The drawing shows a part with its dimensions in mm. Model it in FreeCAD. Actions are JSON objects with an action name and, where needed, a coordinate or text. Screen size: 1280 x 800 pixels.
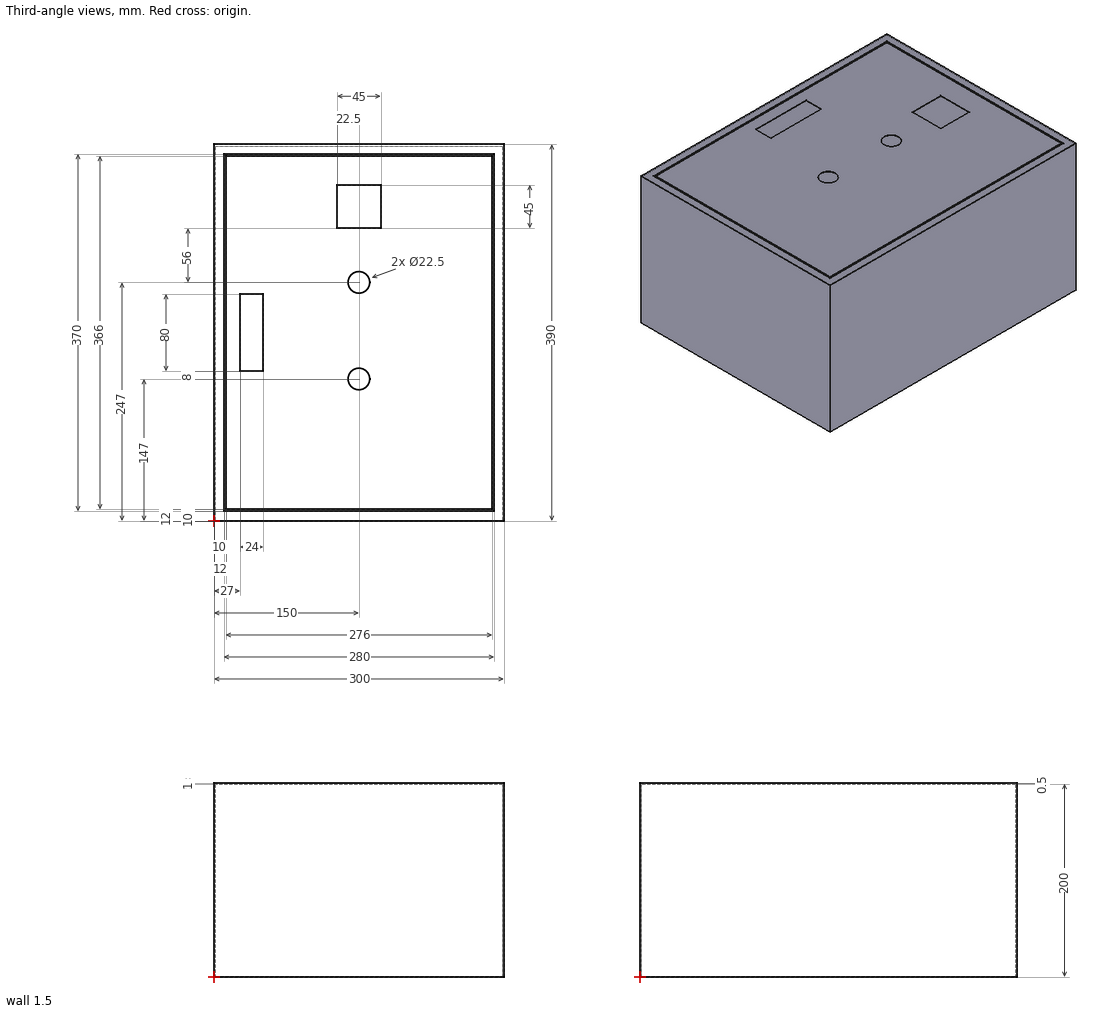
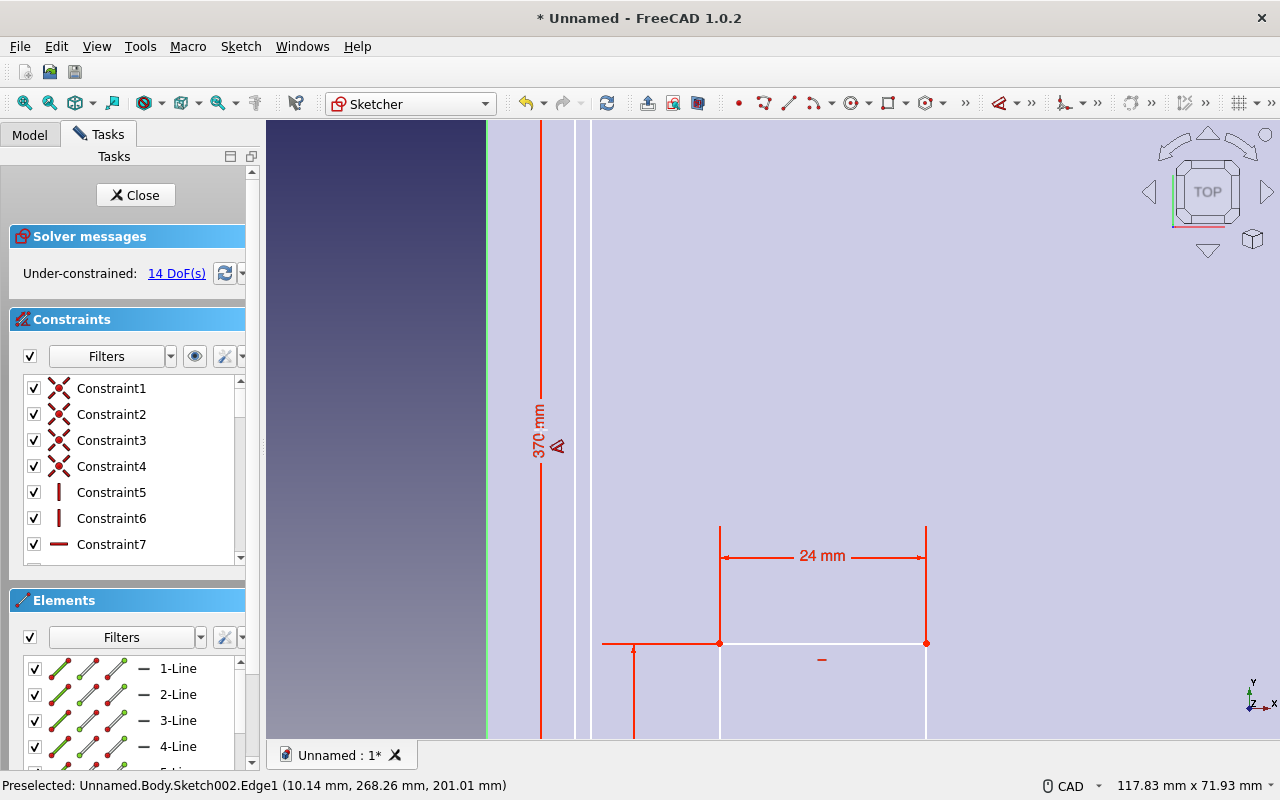
{"action": "scroll", "coordinate": [576, 355], "scroll_direction": "down", "scroll_amount": 11}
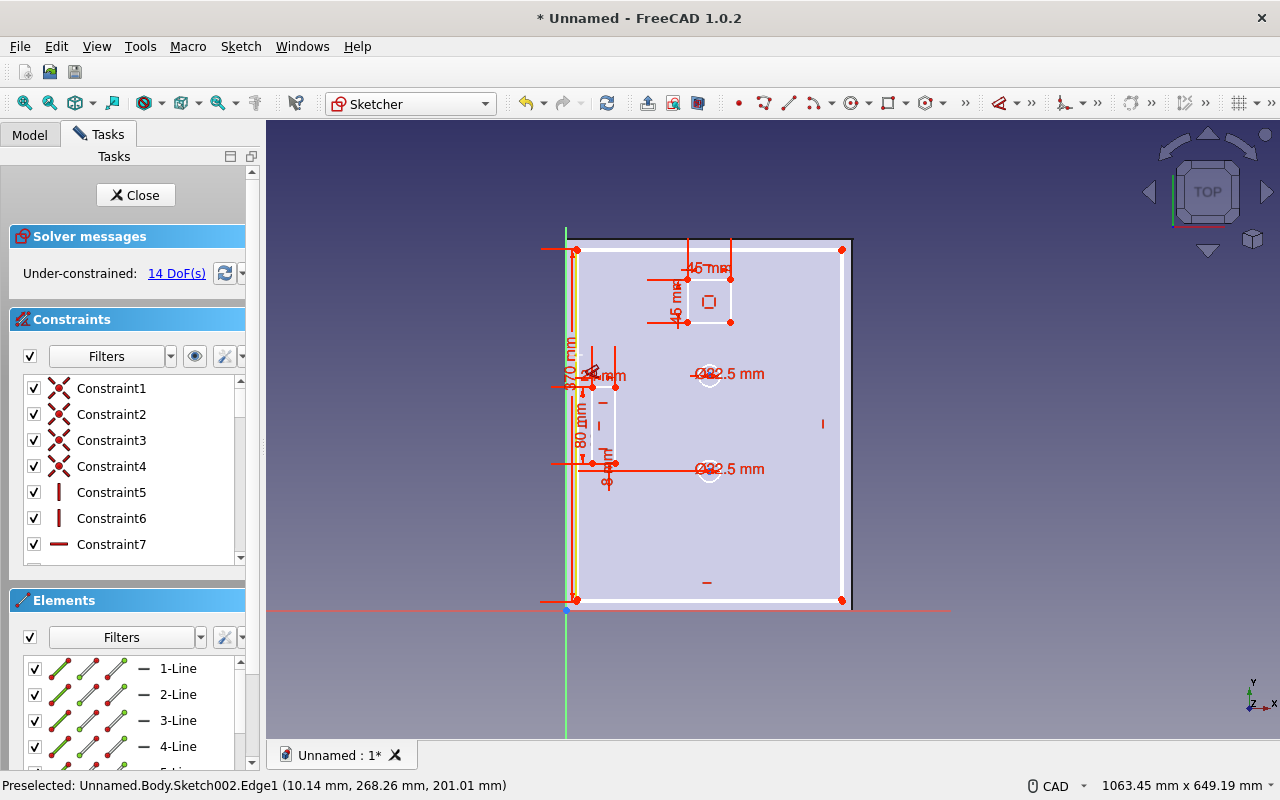
{"action": "scroll", "coordinate": [656, 602], "scroll_direction": "up", "scroll_amount": 9}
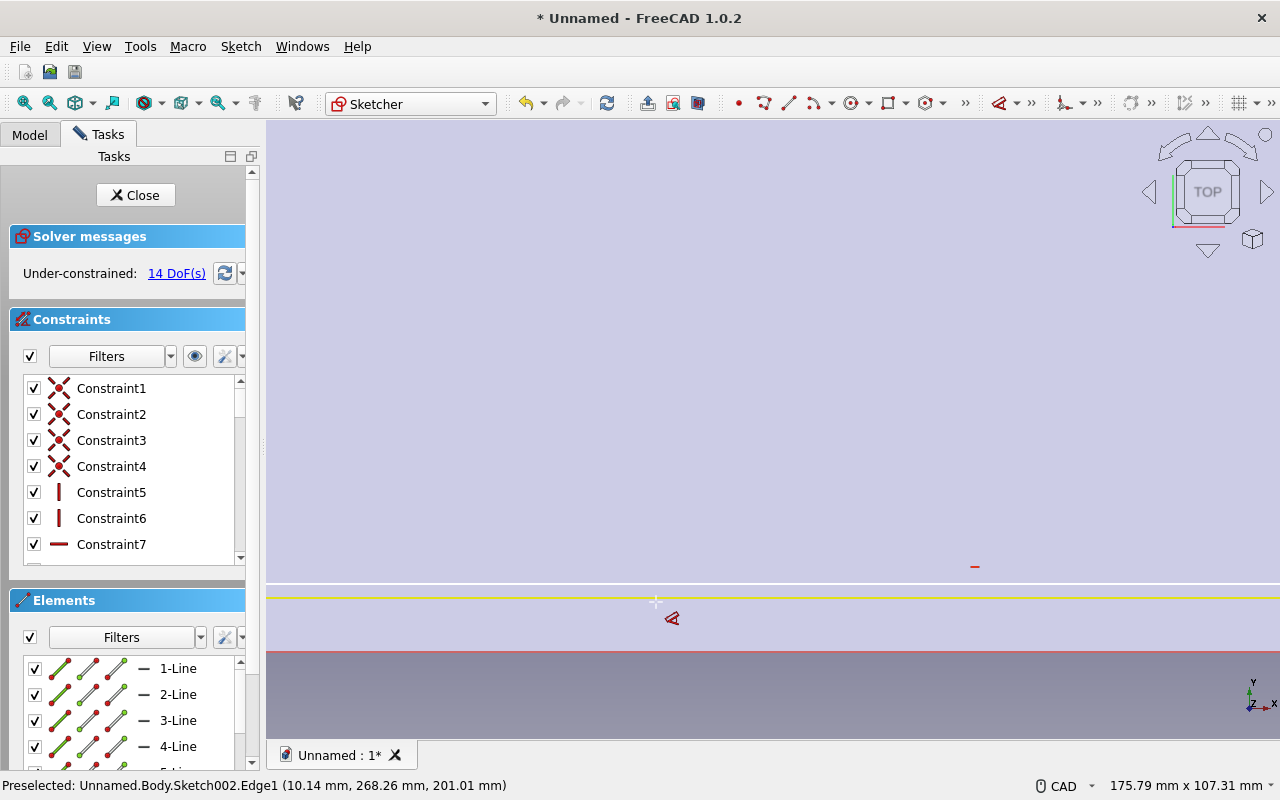
{"action": "left_click", "coordinate": [655, 598]}
{"action": "left_click", "coordinate": [704, 632]}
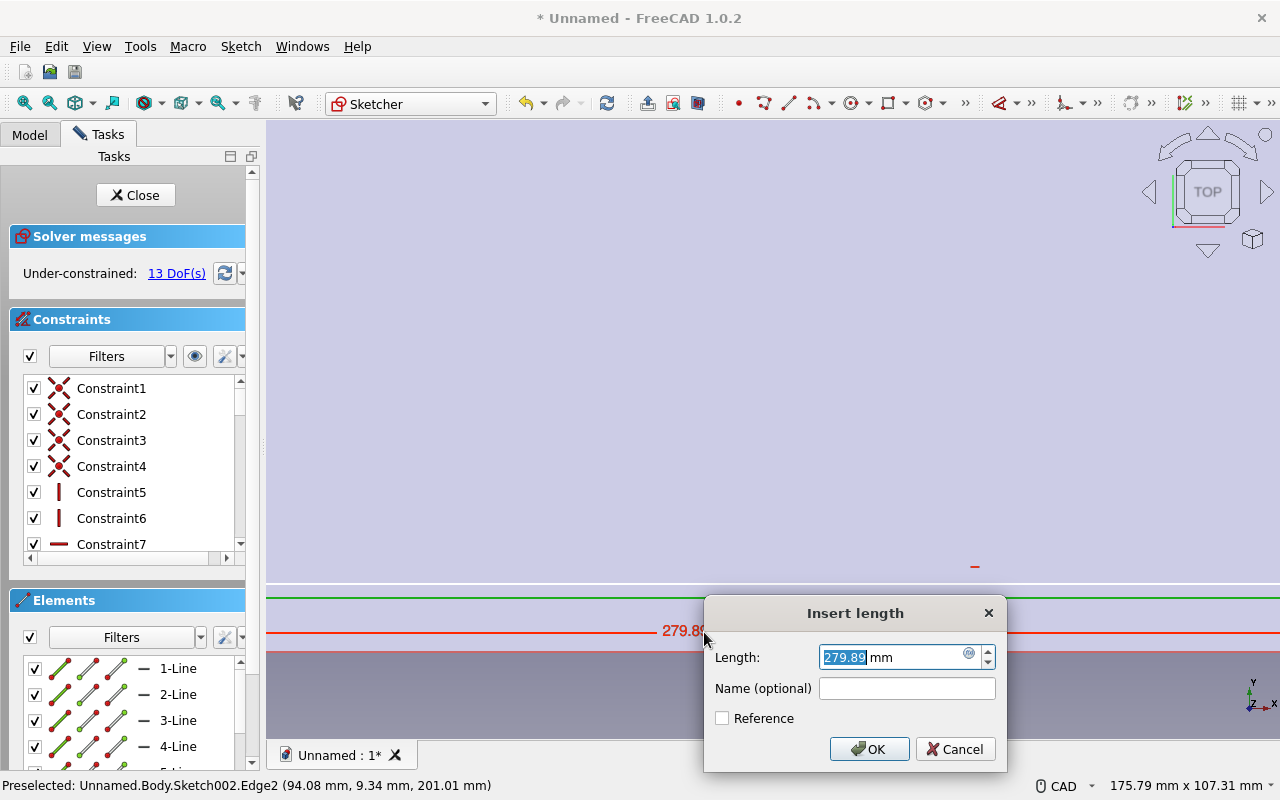
{"action": "type", "text": "280"}
{"action": "key", "text": "Return"}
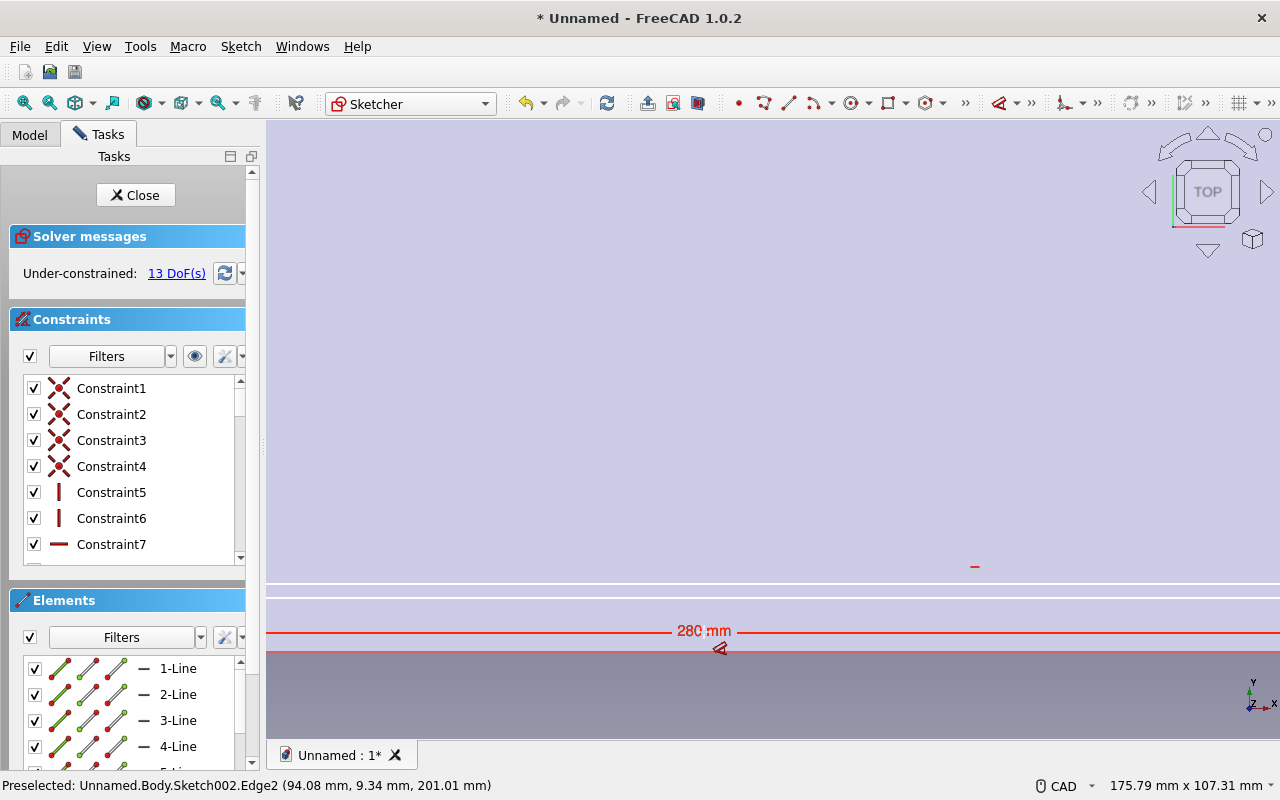
{"action": "scroll", "coordinate": [656, 603], "scroll_direction": "down", "scroll_amount": 9}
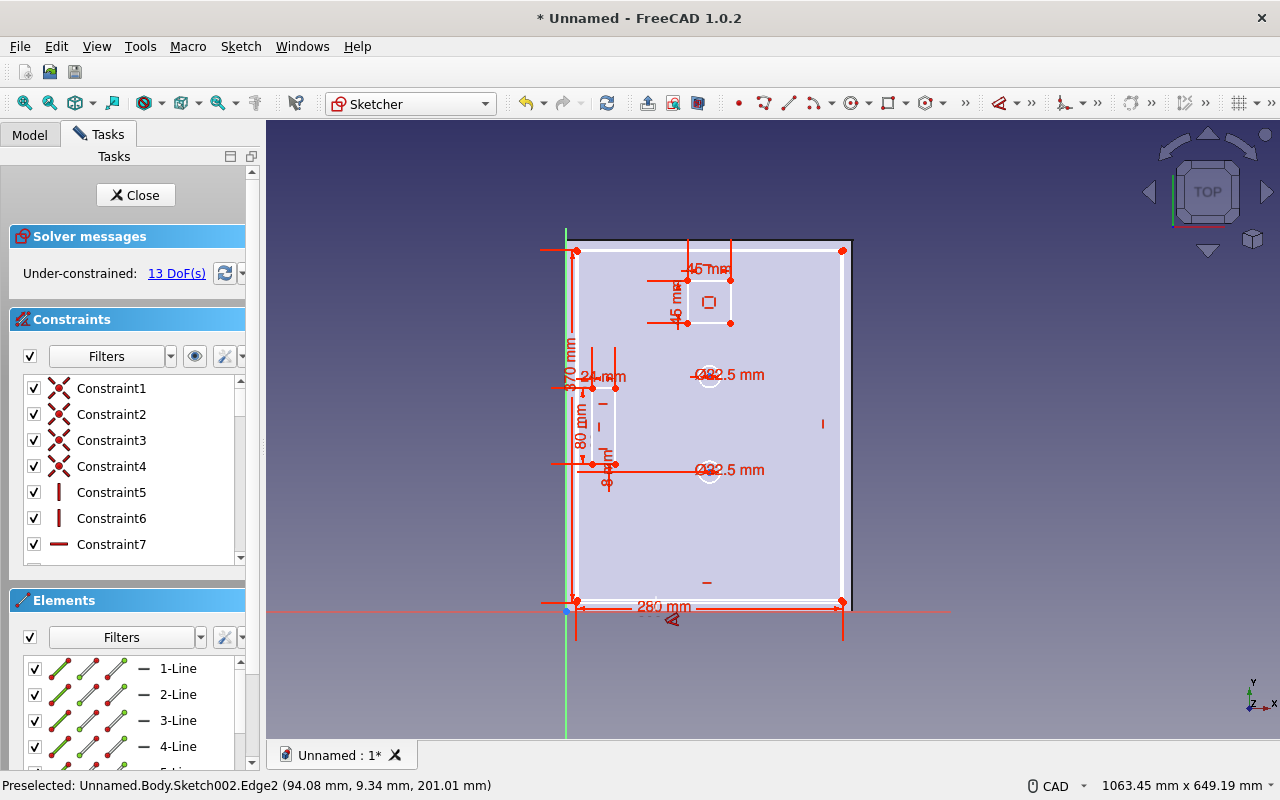
{"action": "scroll", "coordinate": [578, 356], "scroll_direction": "up", "scroll_amount": 11}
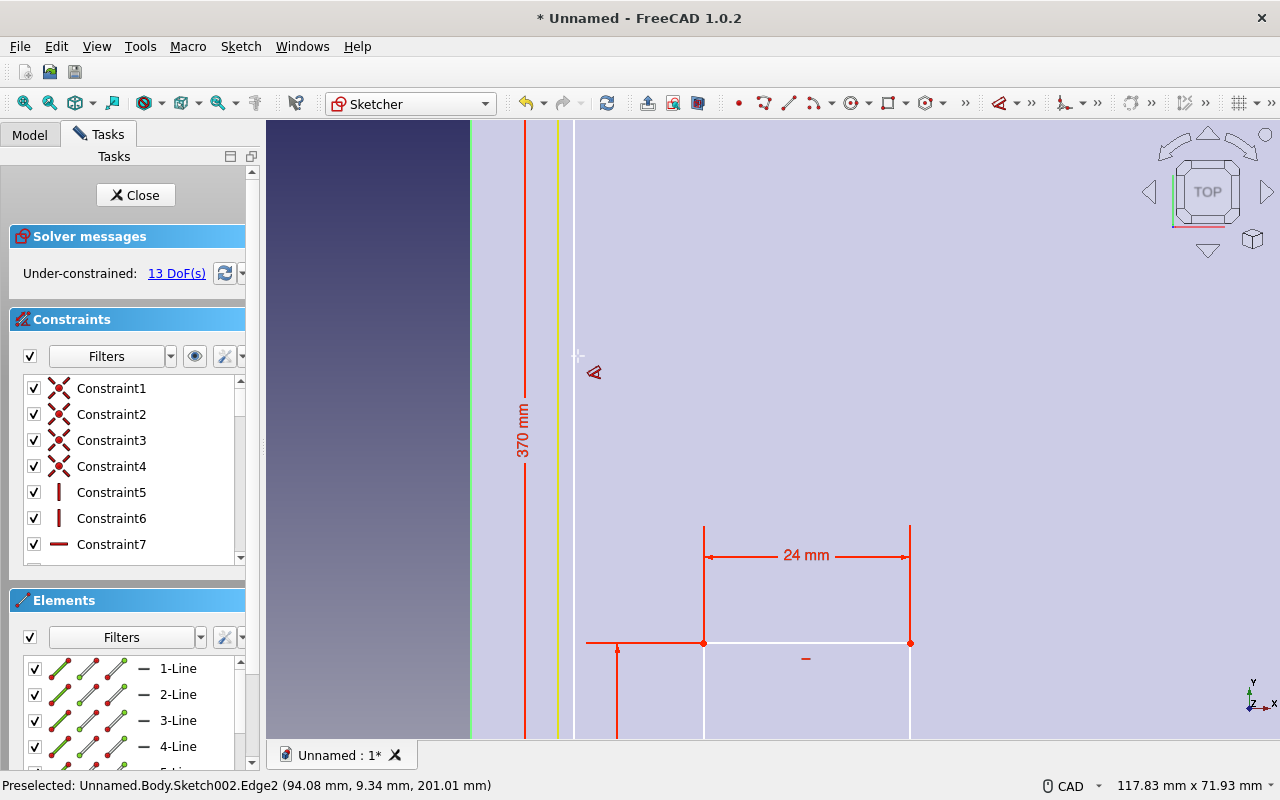
{"action": "left_click", "coordinate": [574, 354]}
{"action": "left_click", "coordinate": [540, 300]}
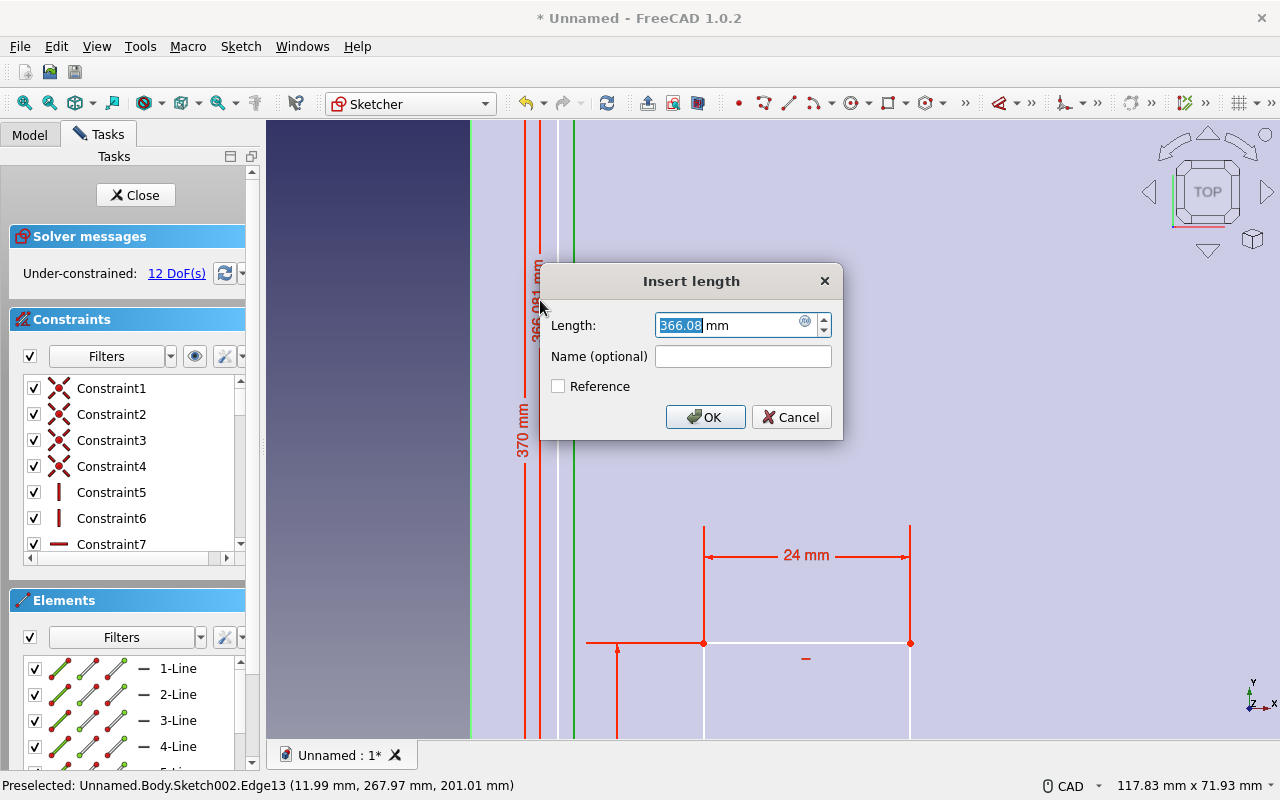
{"action": "type", "text": "366"}
{"action": "key", "text": "Return"}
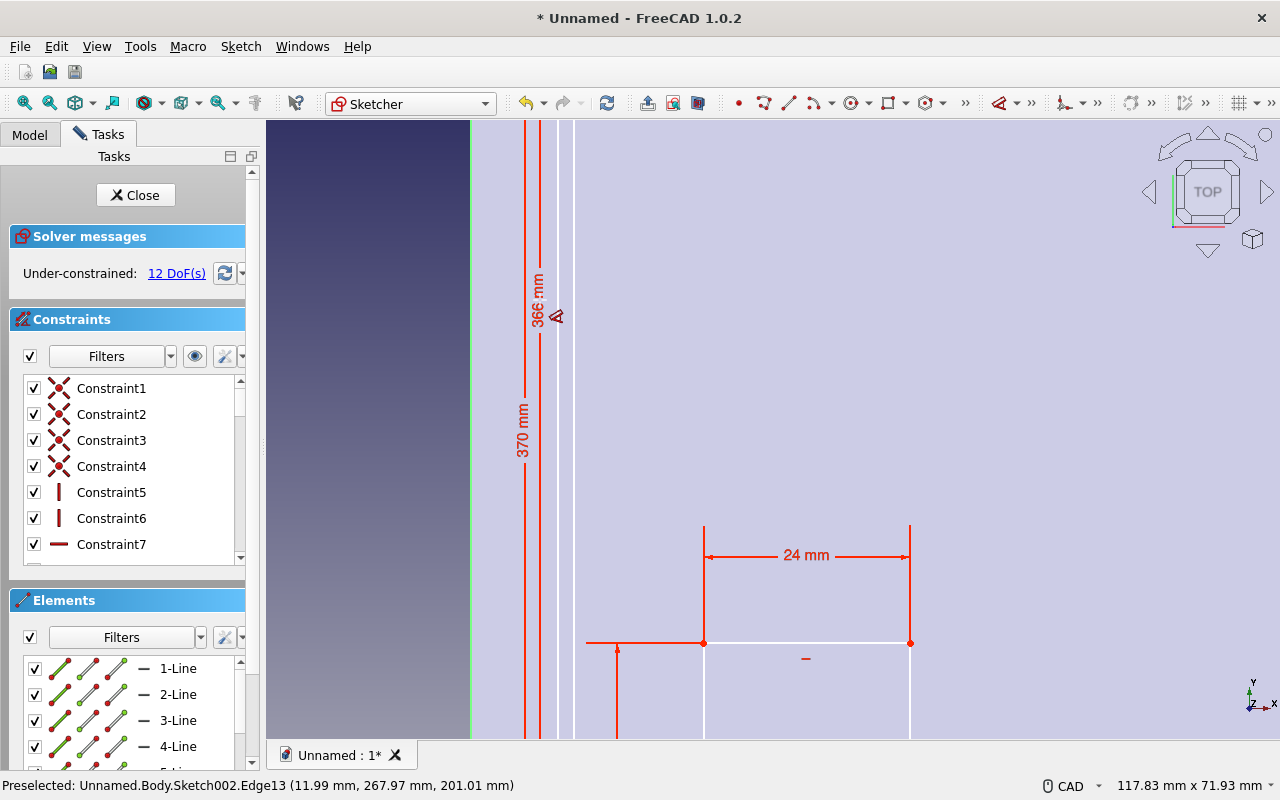
{"action": "scroll", "coordinate": [578, 355], "scroll_direction": "down", "scroll_amount": 11}